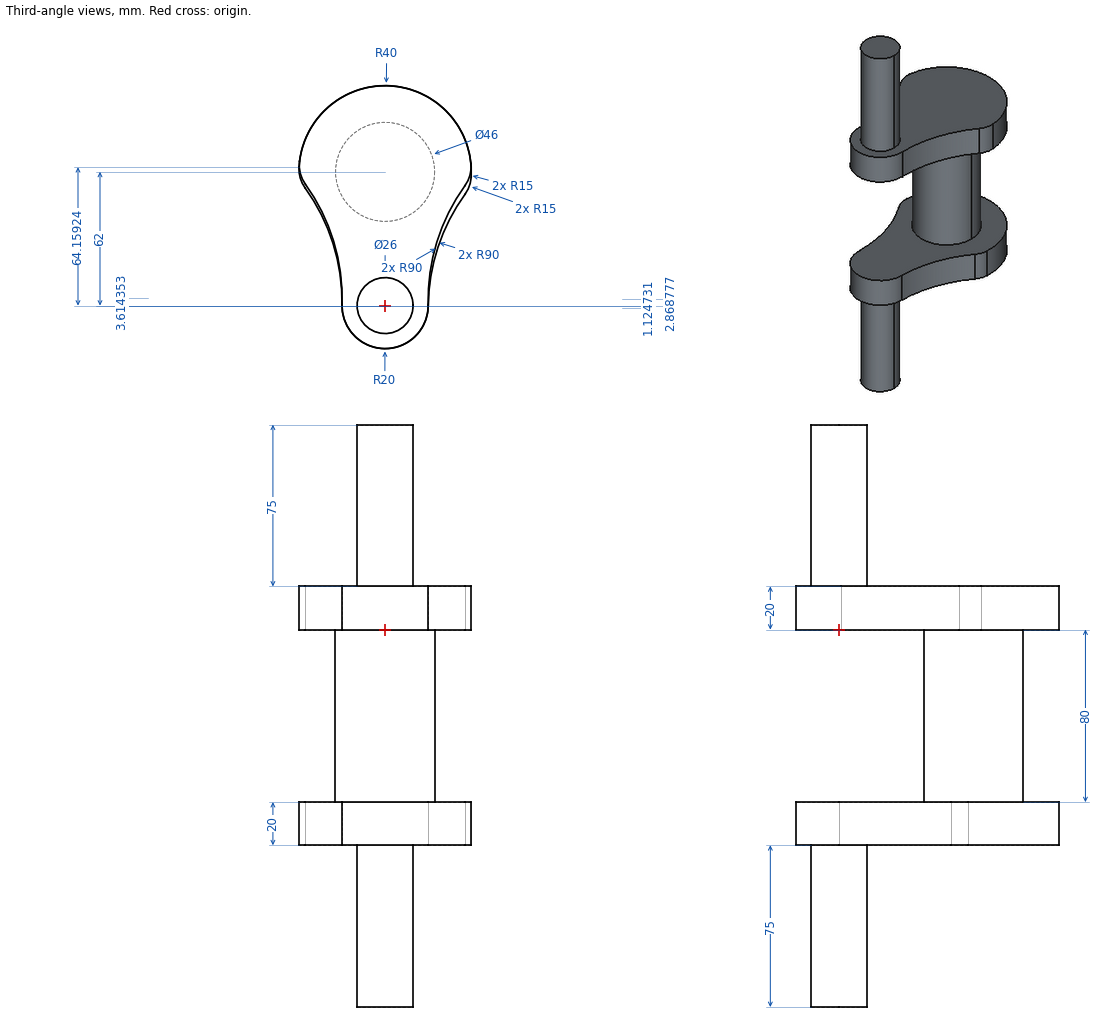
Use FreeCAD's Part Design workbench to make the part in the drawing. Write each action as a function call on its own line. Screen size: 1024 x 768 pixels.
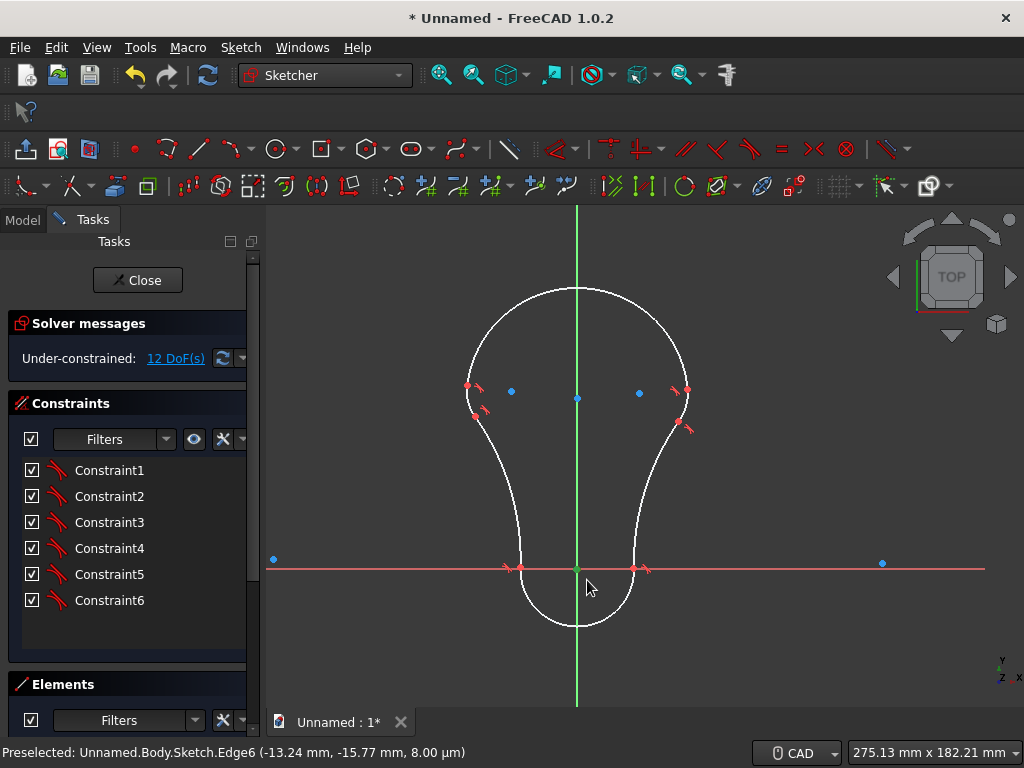
click(610, 150)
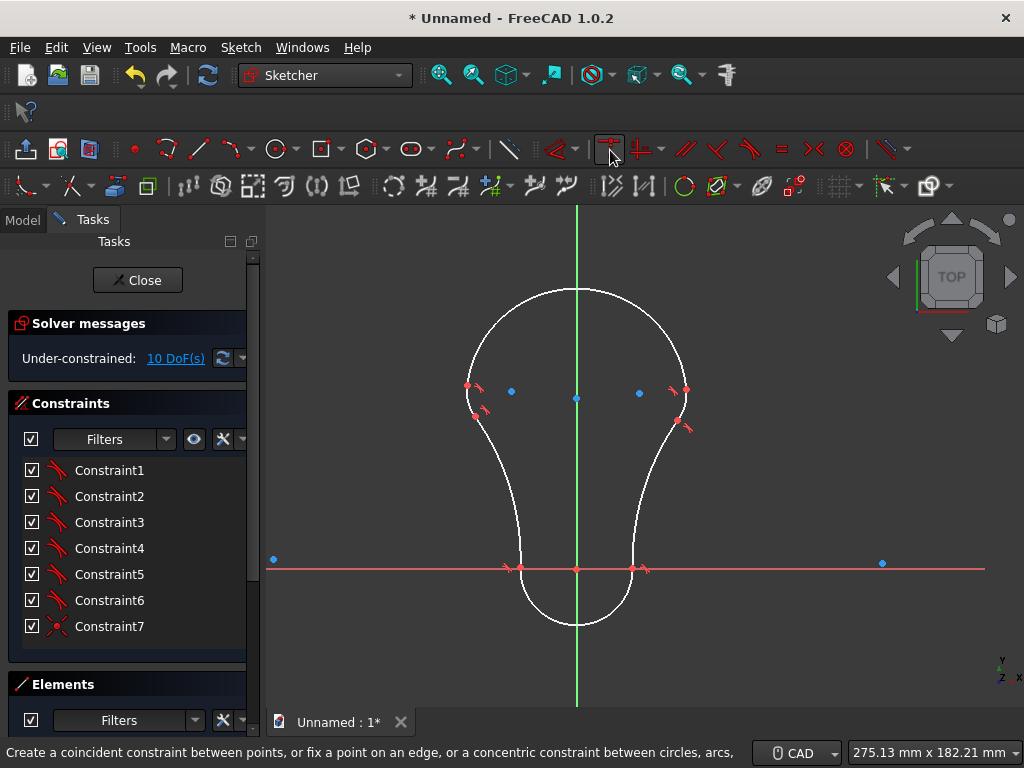
scroll(683, 412, up, 2)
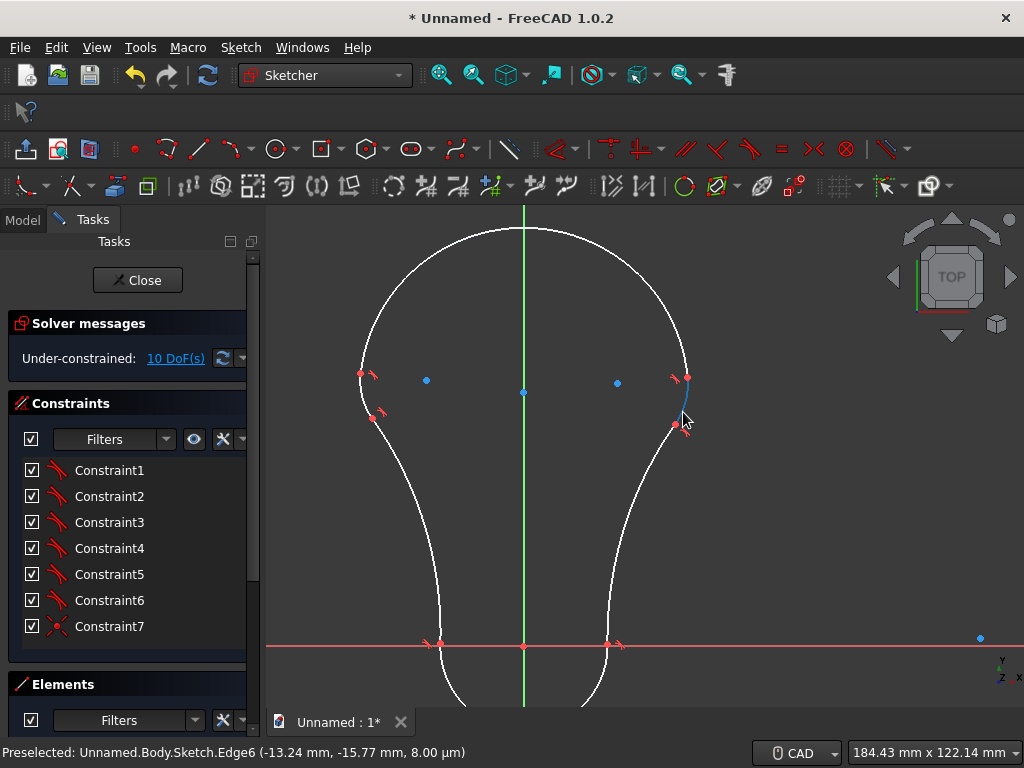
click(682, 411)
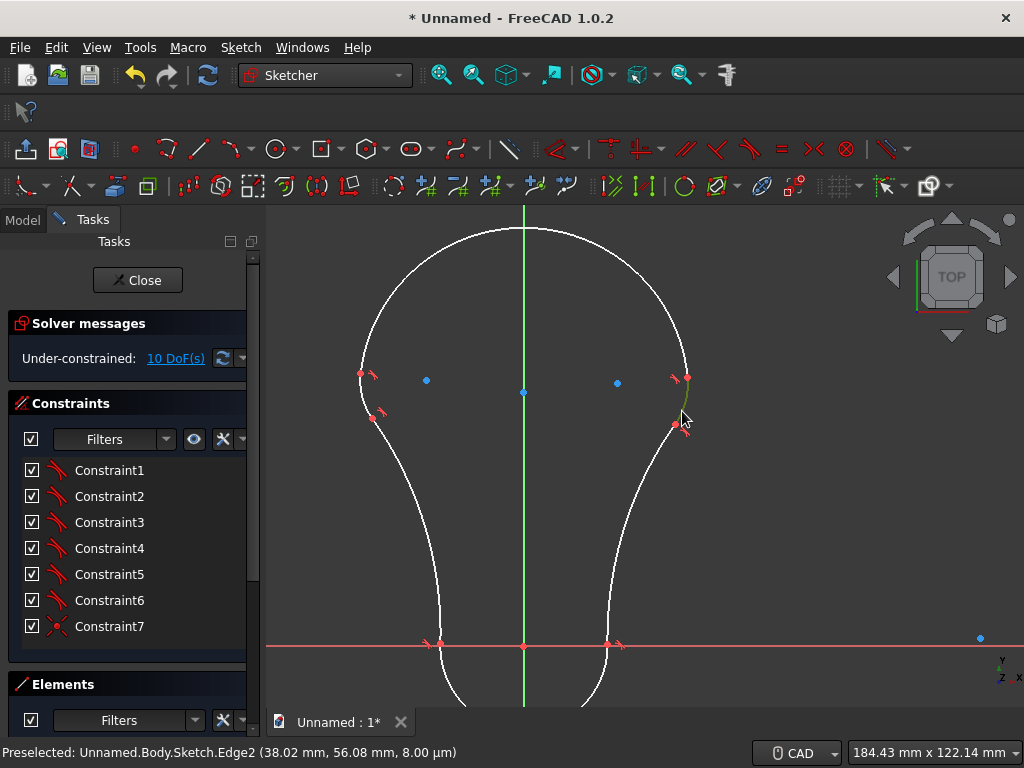
click(361, 387)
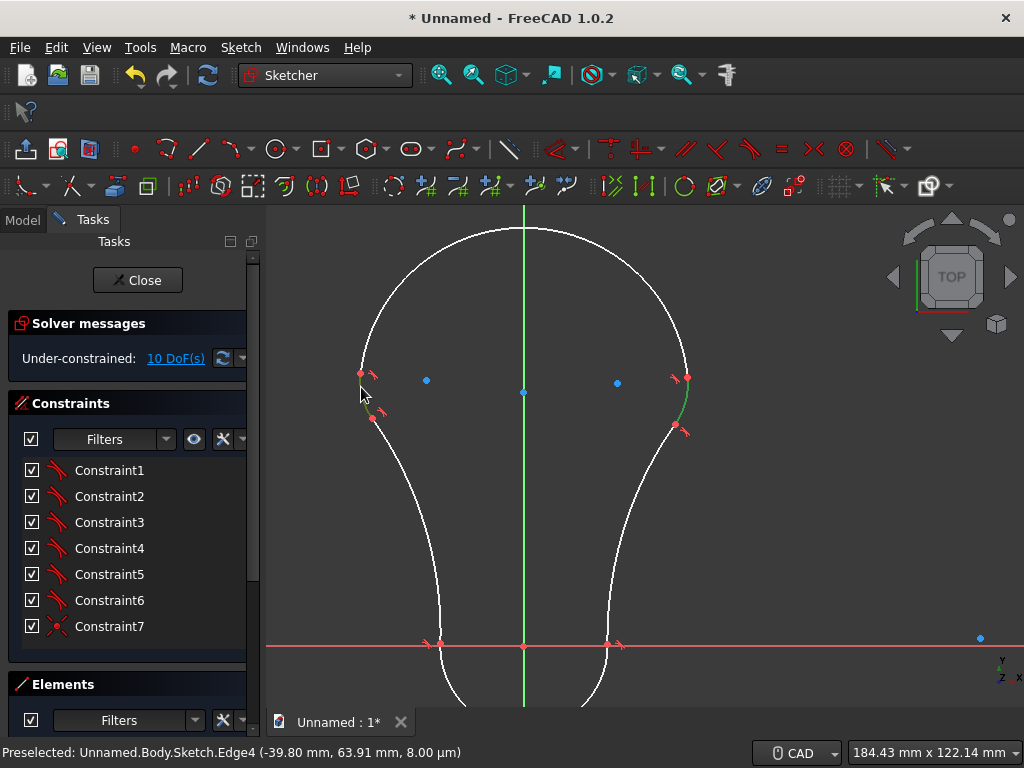
click(782, 150)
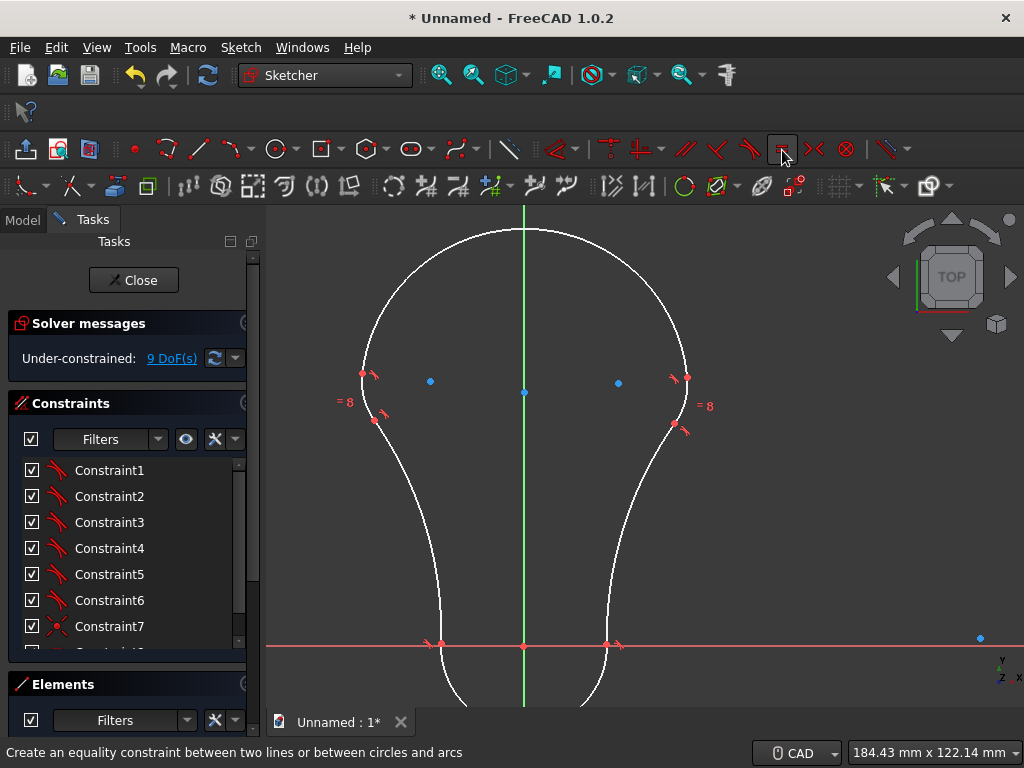
click(640, 485)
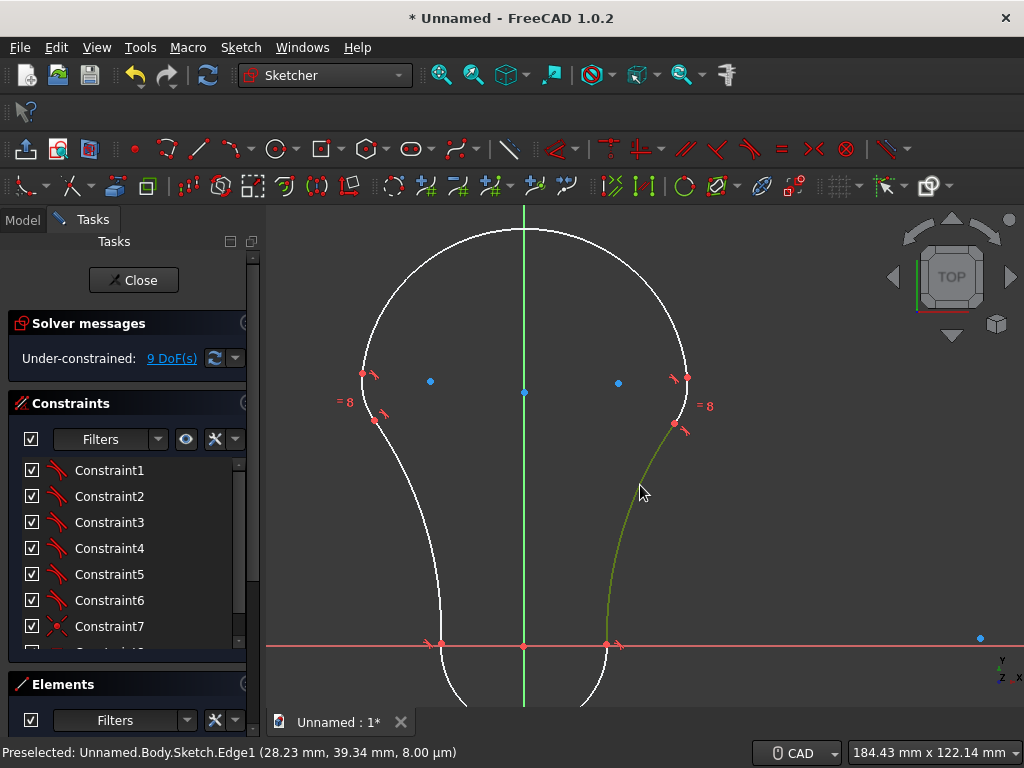
click(436, 573)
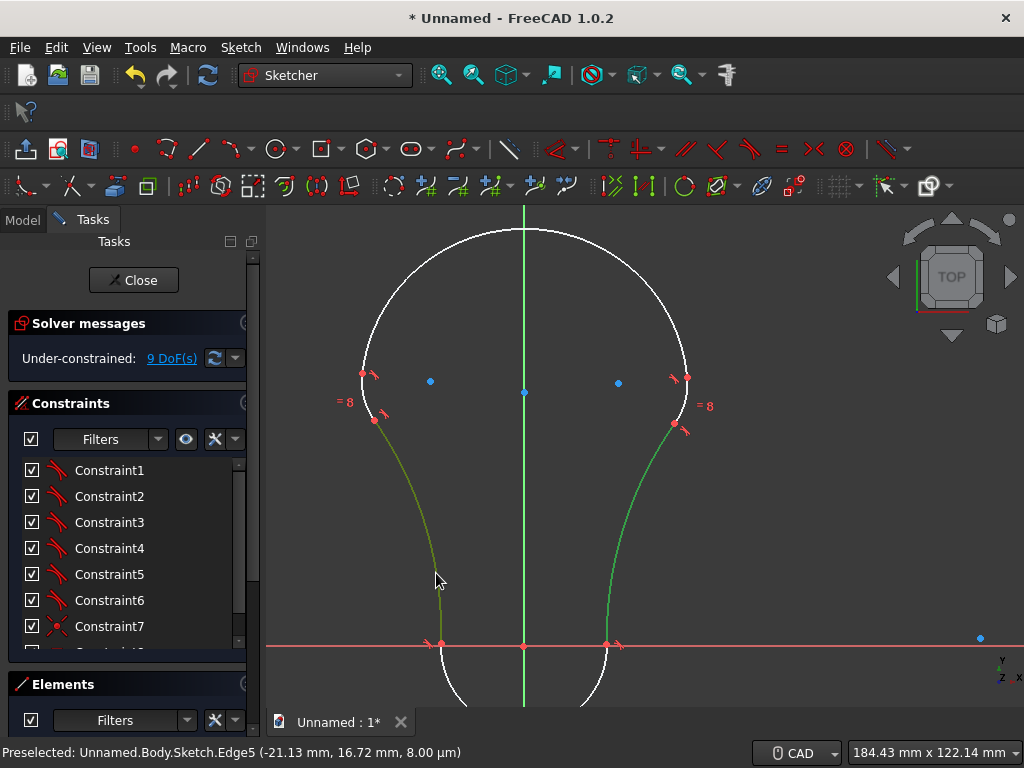
click(782, 150)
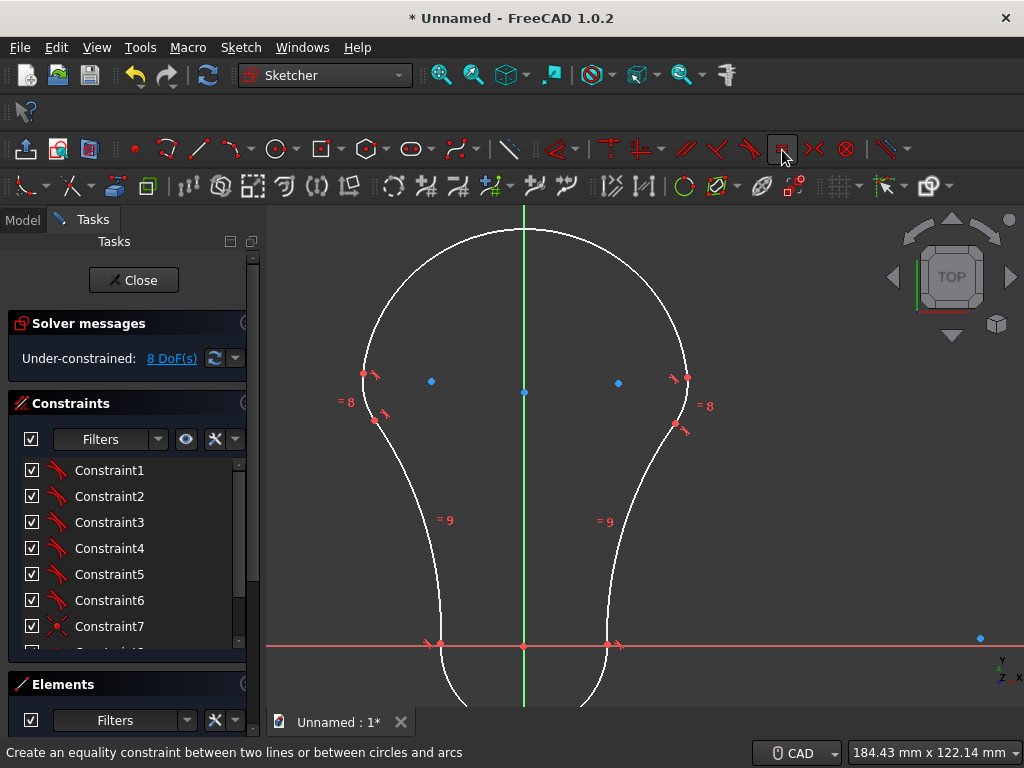
click(525, 392)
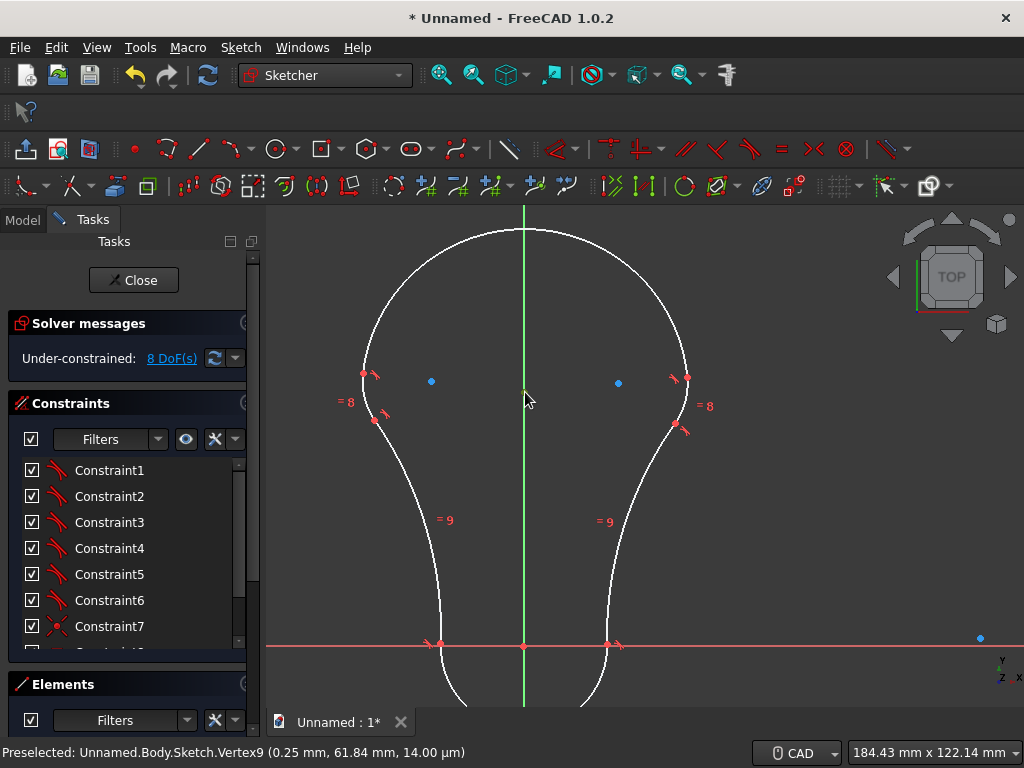
click(524, 615)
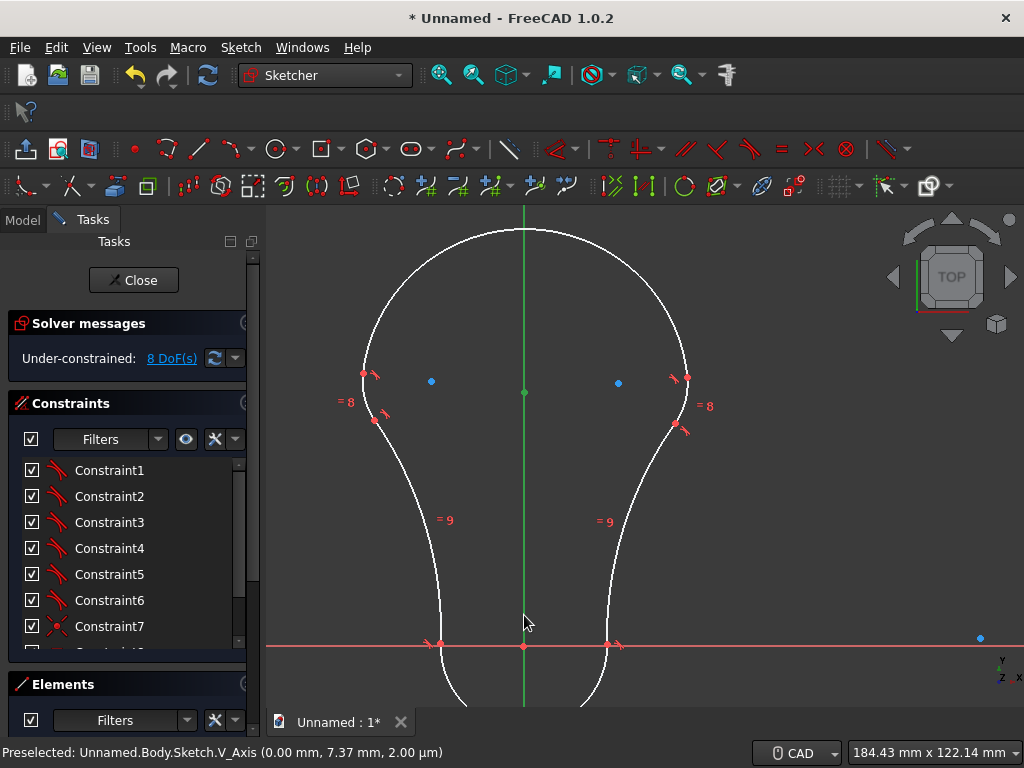
click(610, 150)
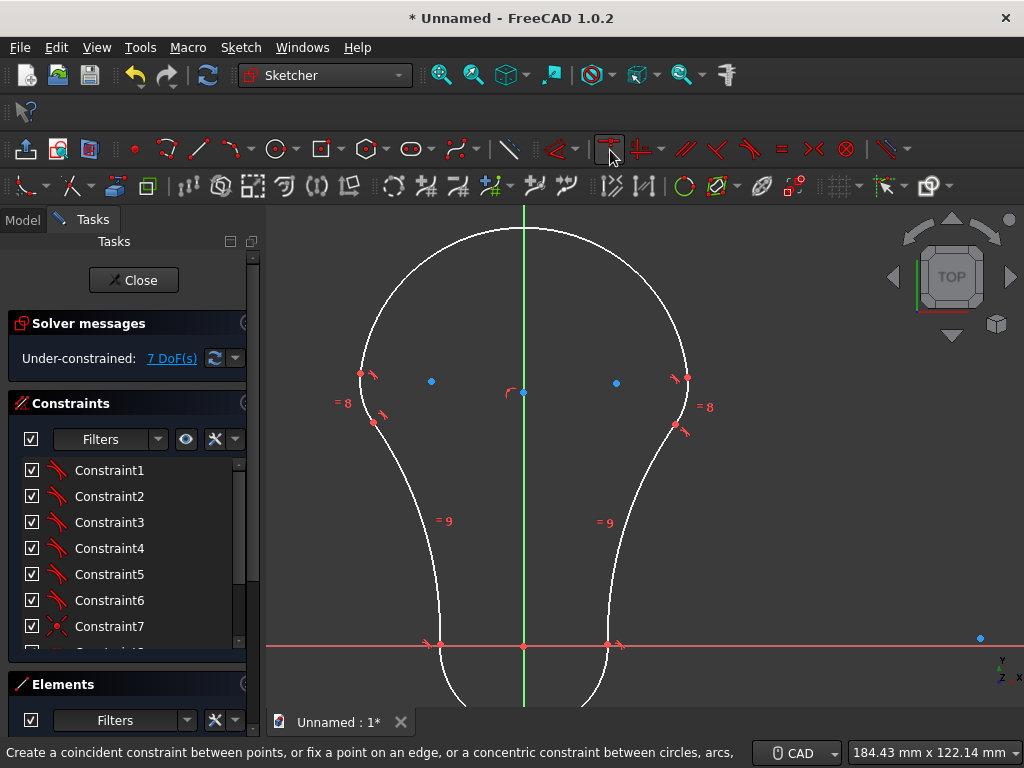
click(640, 486)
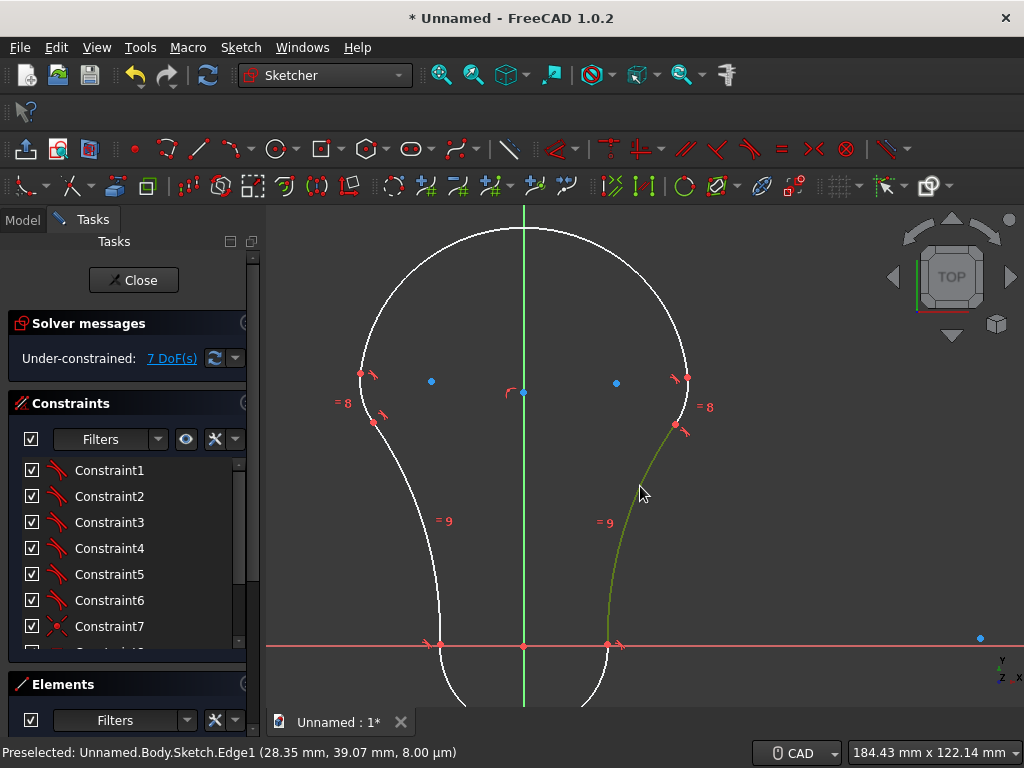
key(k)
key(r)